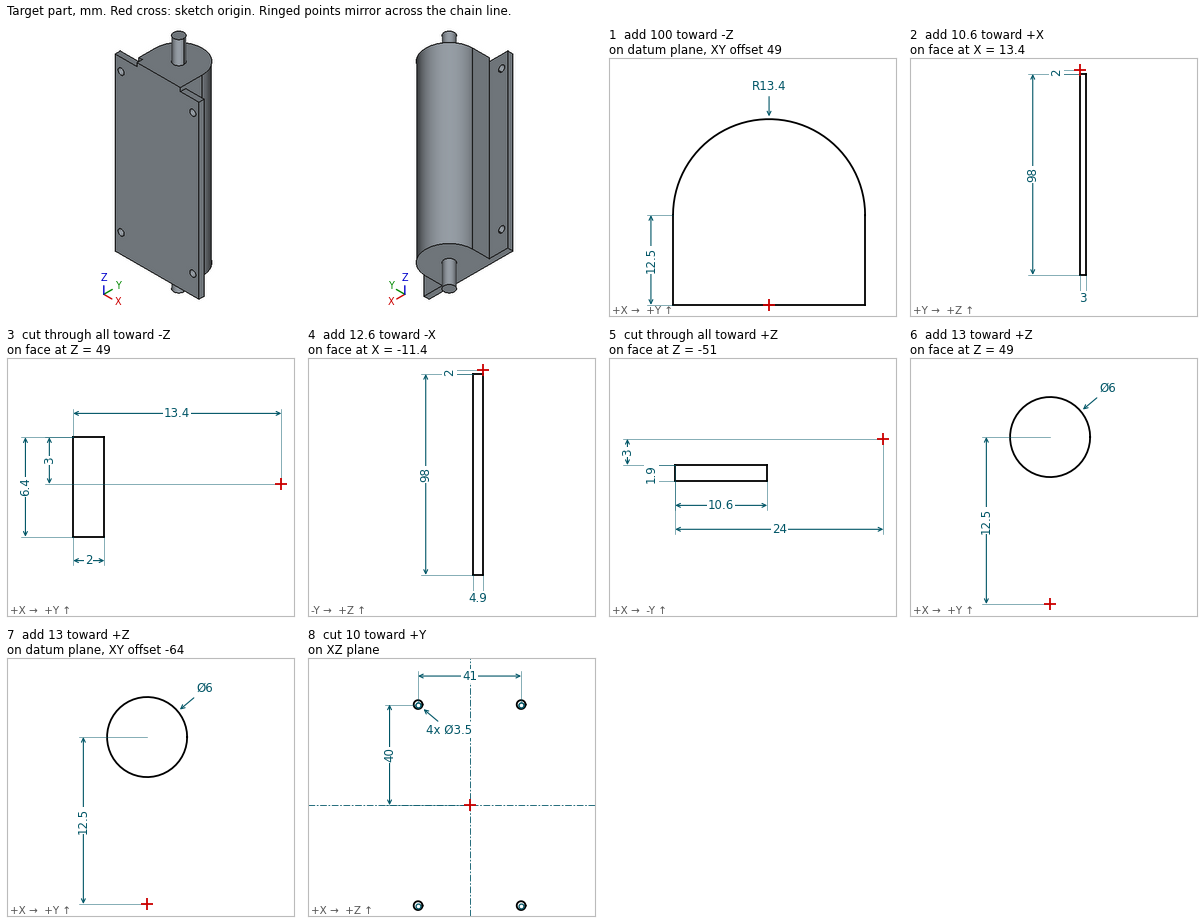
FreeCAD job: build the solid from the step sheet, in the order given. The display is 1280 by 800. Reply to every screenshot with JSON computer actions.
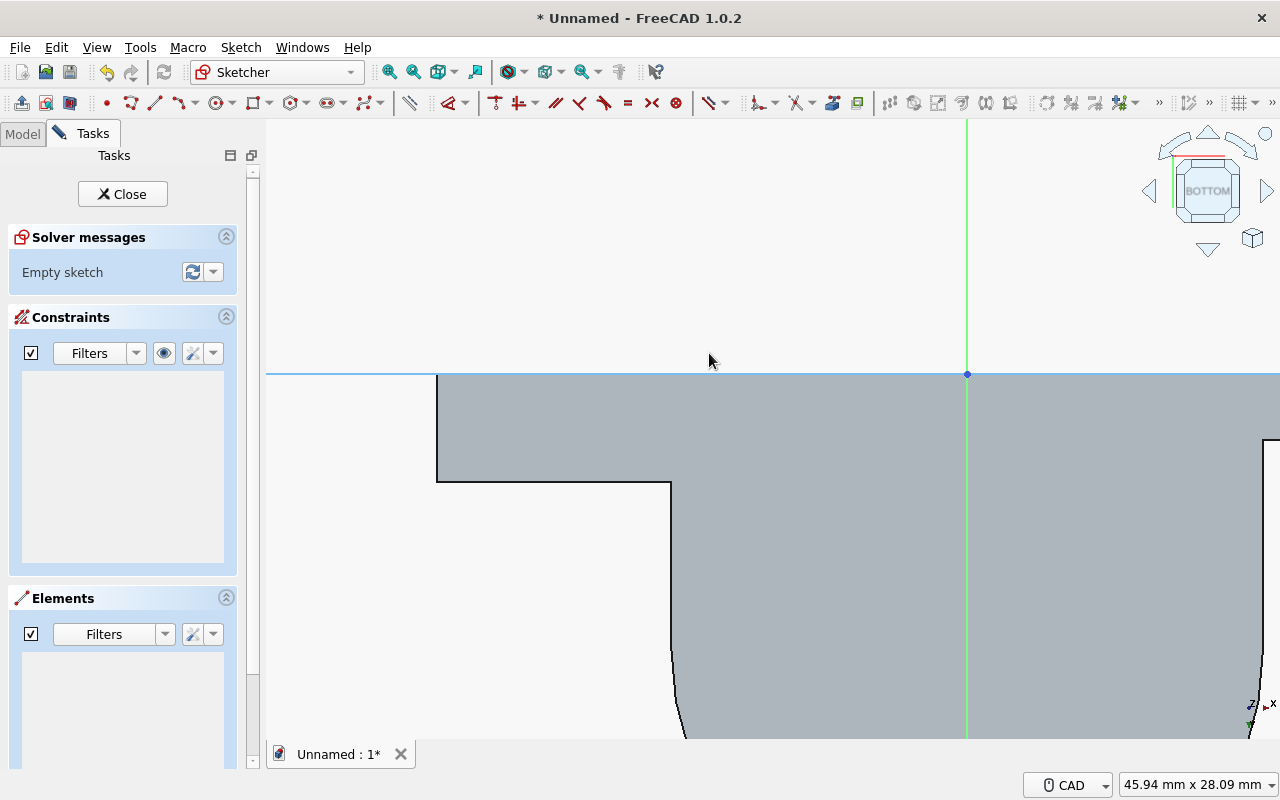
{"action": "left_click", "coordinate": [254, 104]}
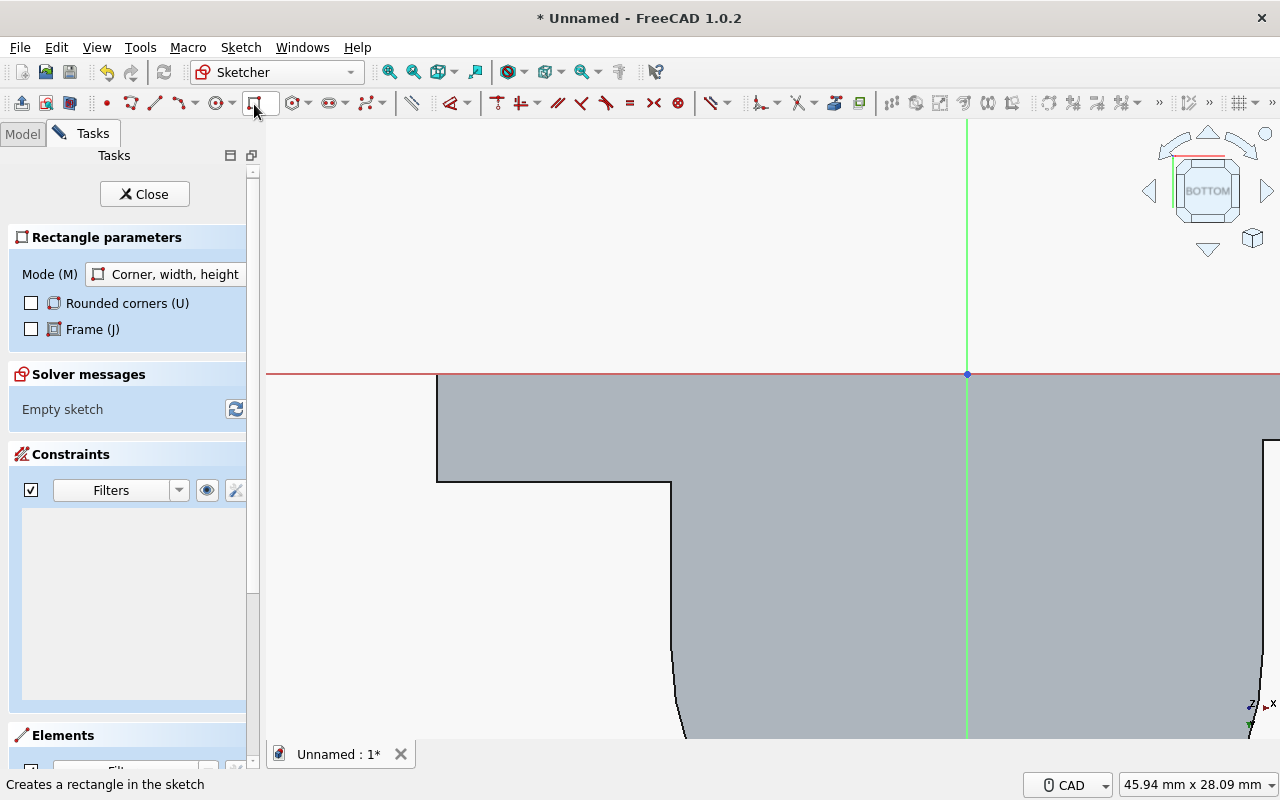
{"action": "left_click", "coordinate": [437, 440]}
{"action": "left_click", "coordinate": [671, 482]}
{"action": "key", "text": "Escape"}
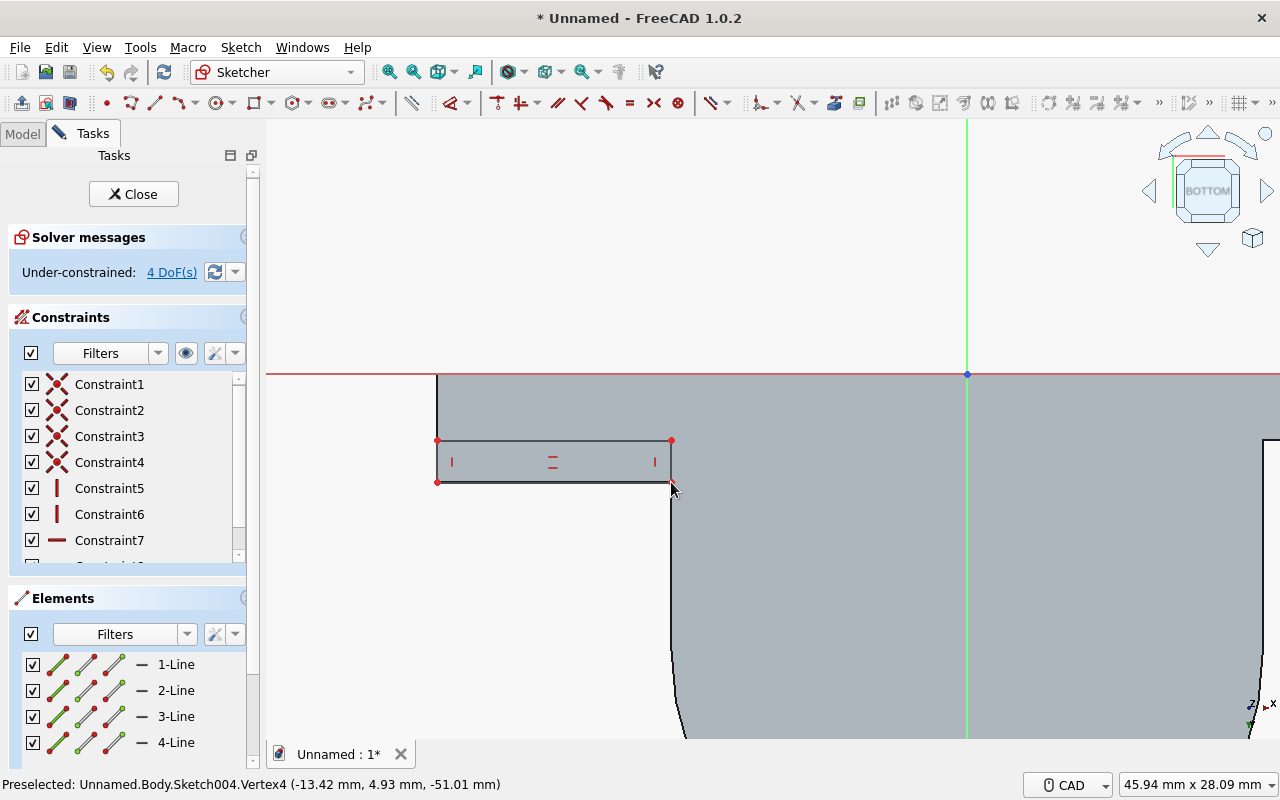
{"action": "left_click", "coordinate": [450, 104]}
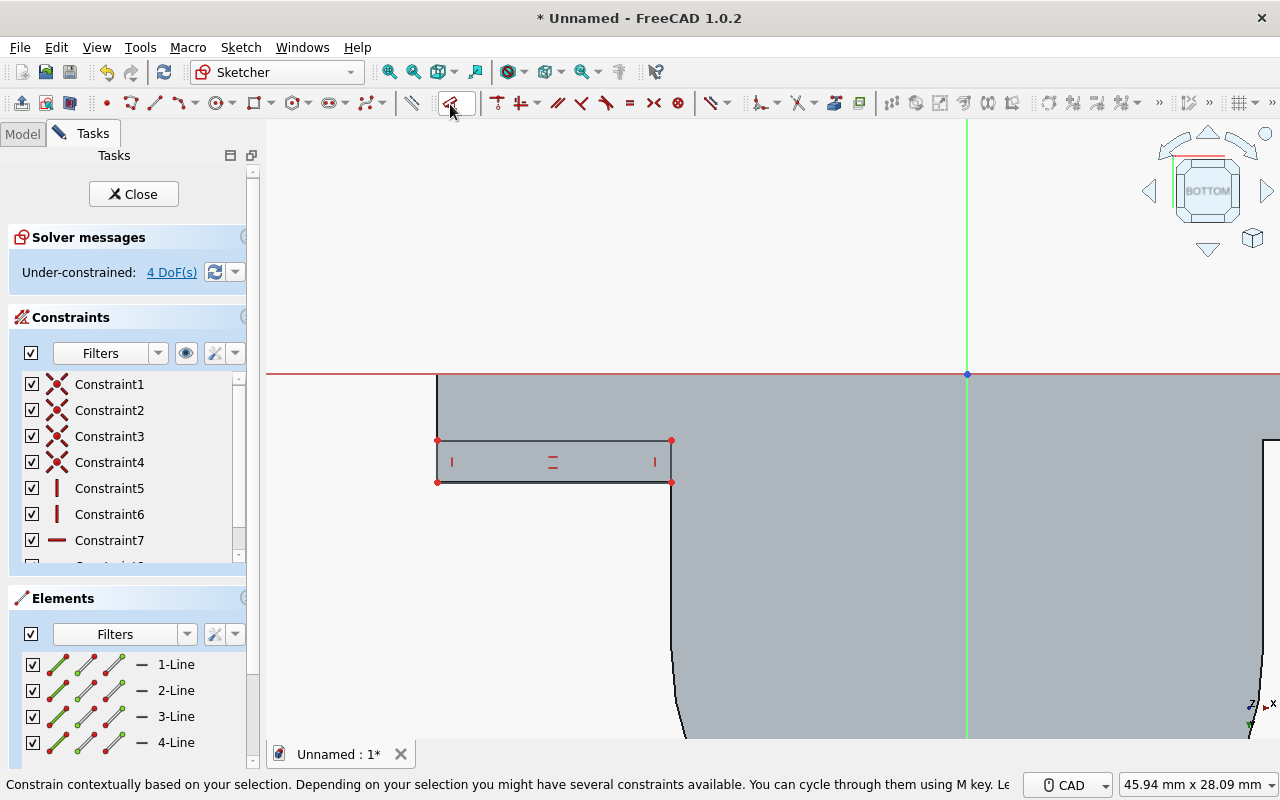
{"action": "left_click", "coordinate": [437, 441]}
{"action": "left_click", "coordinate": [403, 408]}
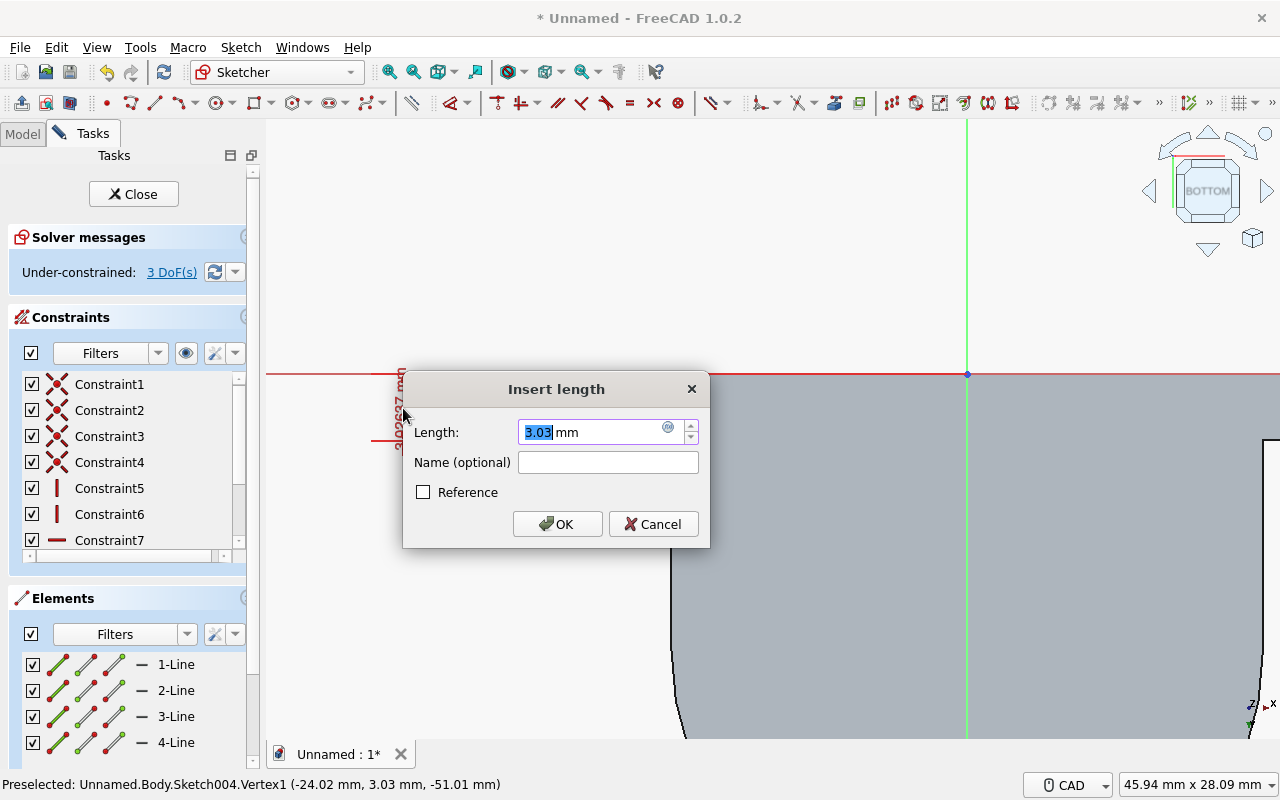
{"action": "type", "text": "3"}
{"action": "key", "text": "Return"}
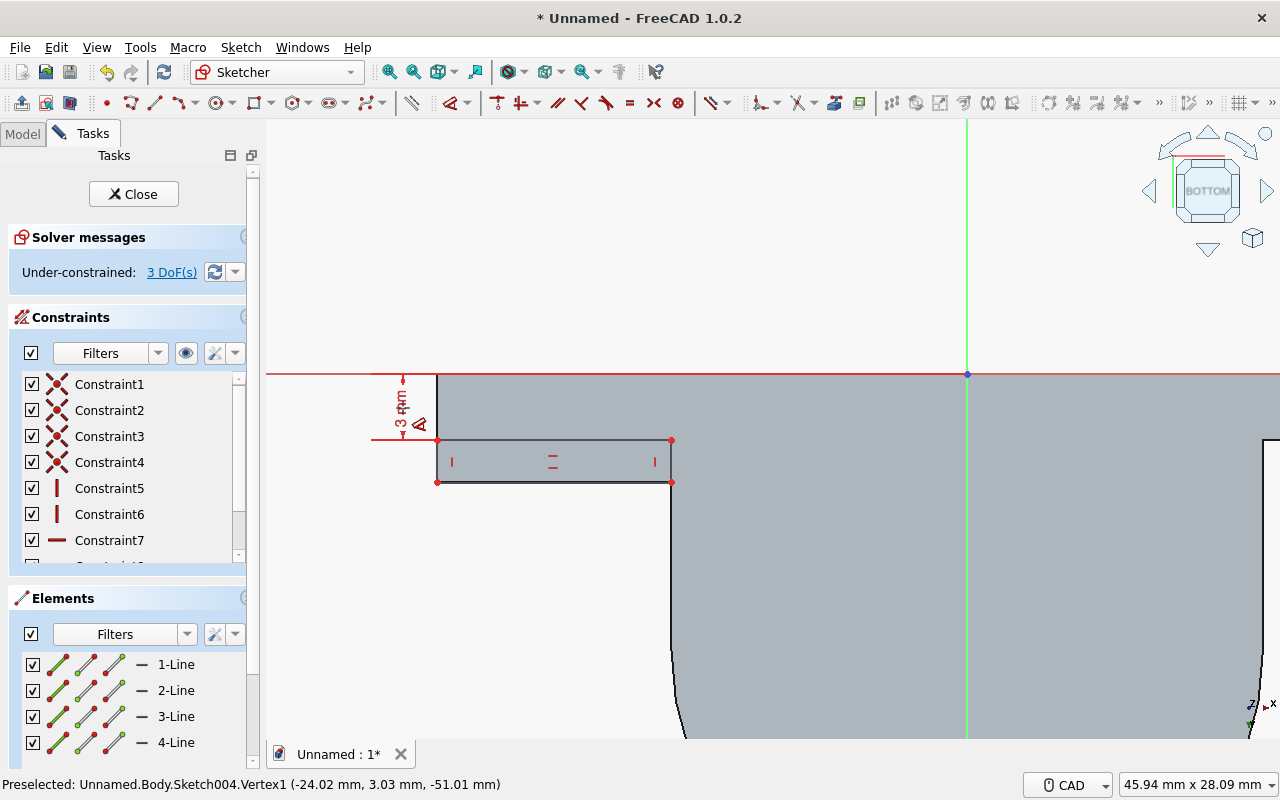
{"action": "left_click", "coordinate": [437, 453]}
{"action": "left_click", "coordinate": [403, 462]}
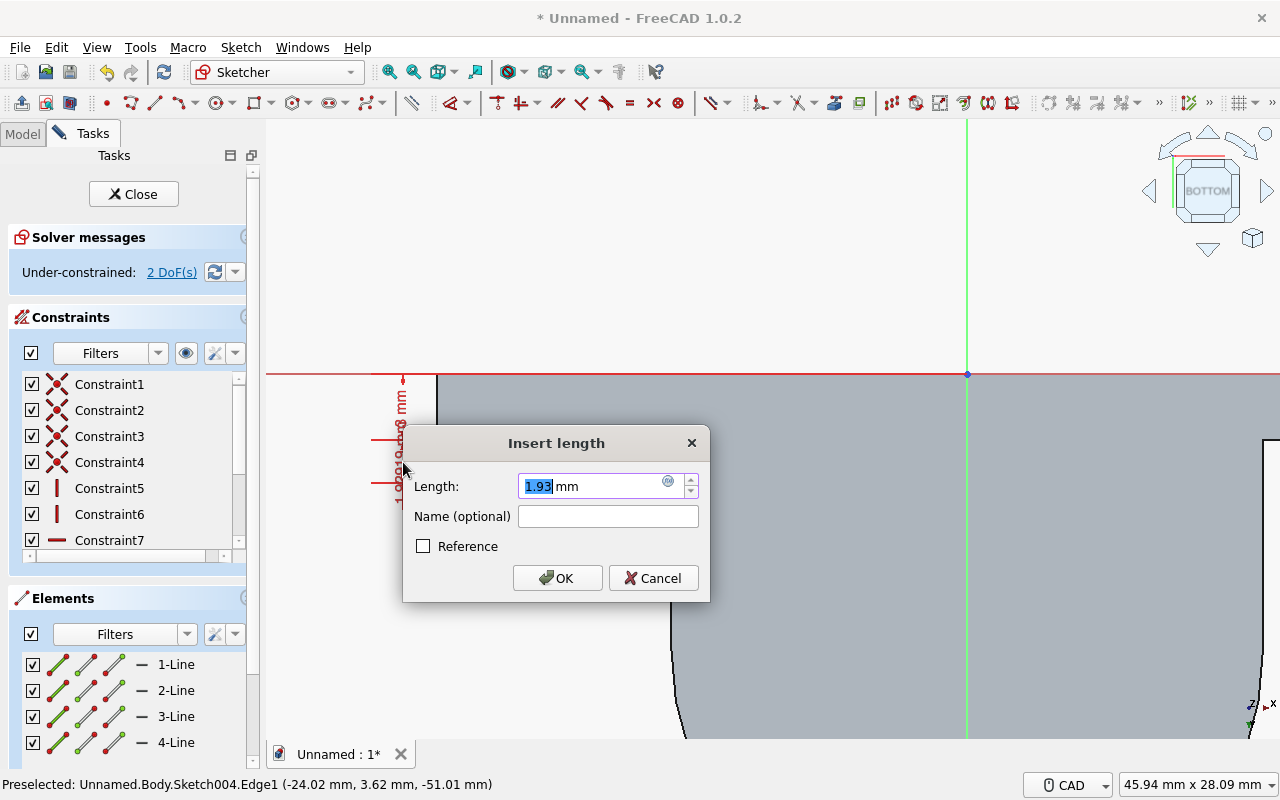
{"action": "type", "text": "1.9"}
{"action": "key", "text": "Return"}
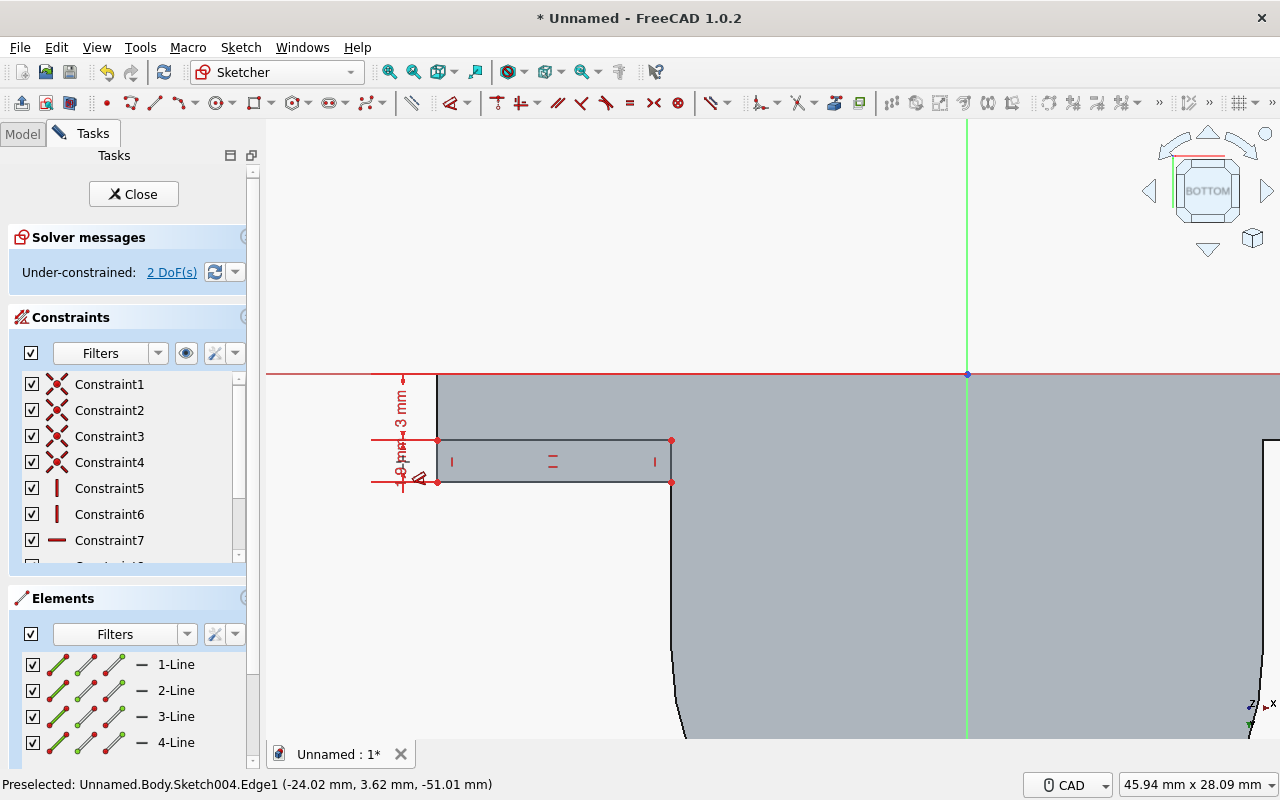
{"action": "left_click", "coordinate": [437, 440]}
{"action": "left_click", "coordinate": [702, 340]}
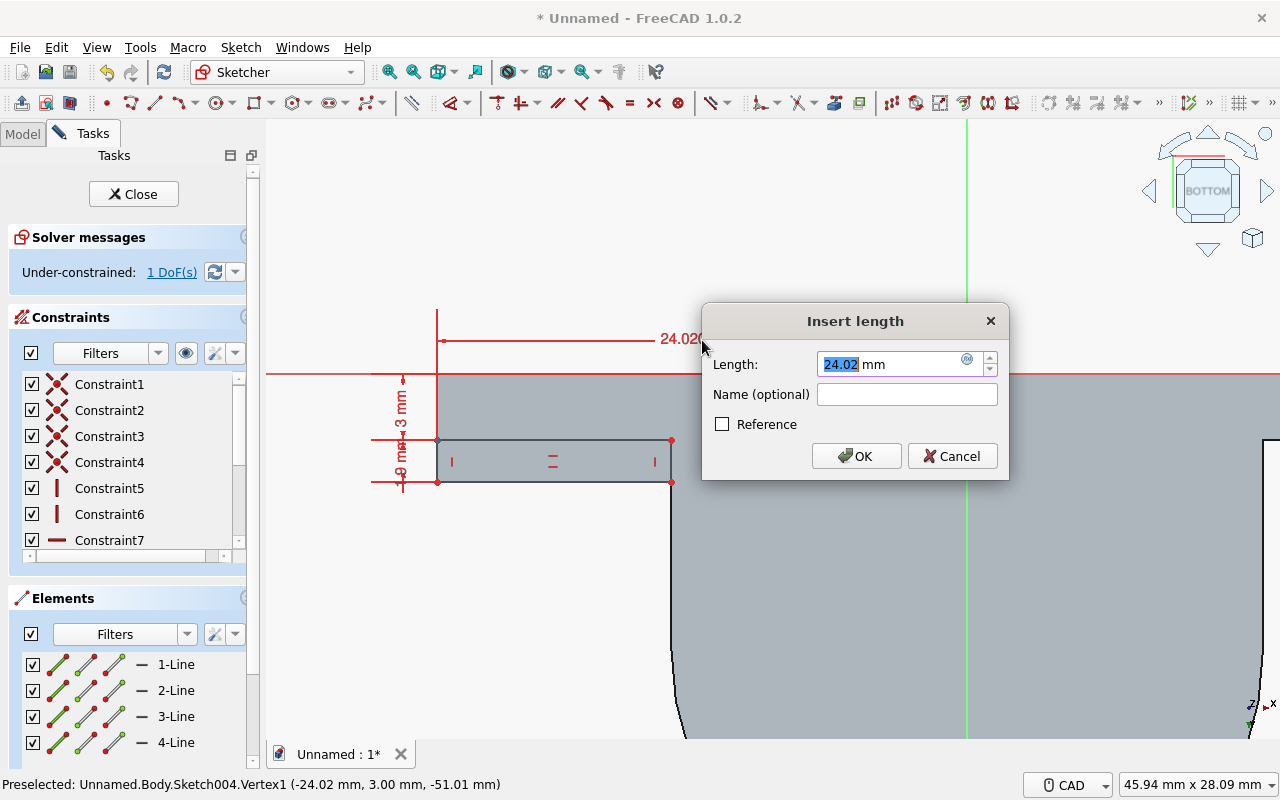
{"action": "type", "text": "24"}
{"action": "key", "text": "Return"}